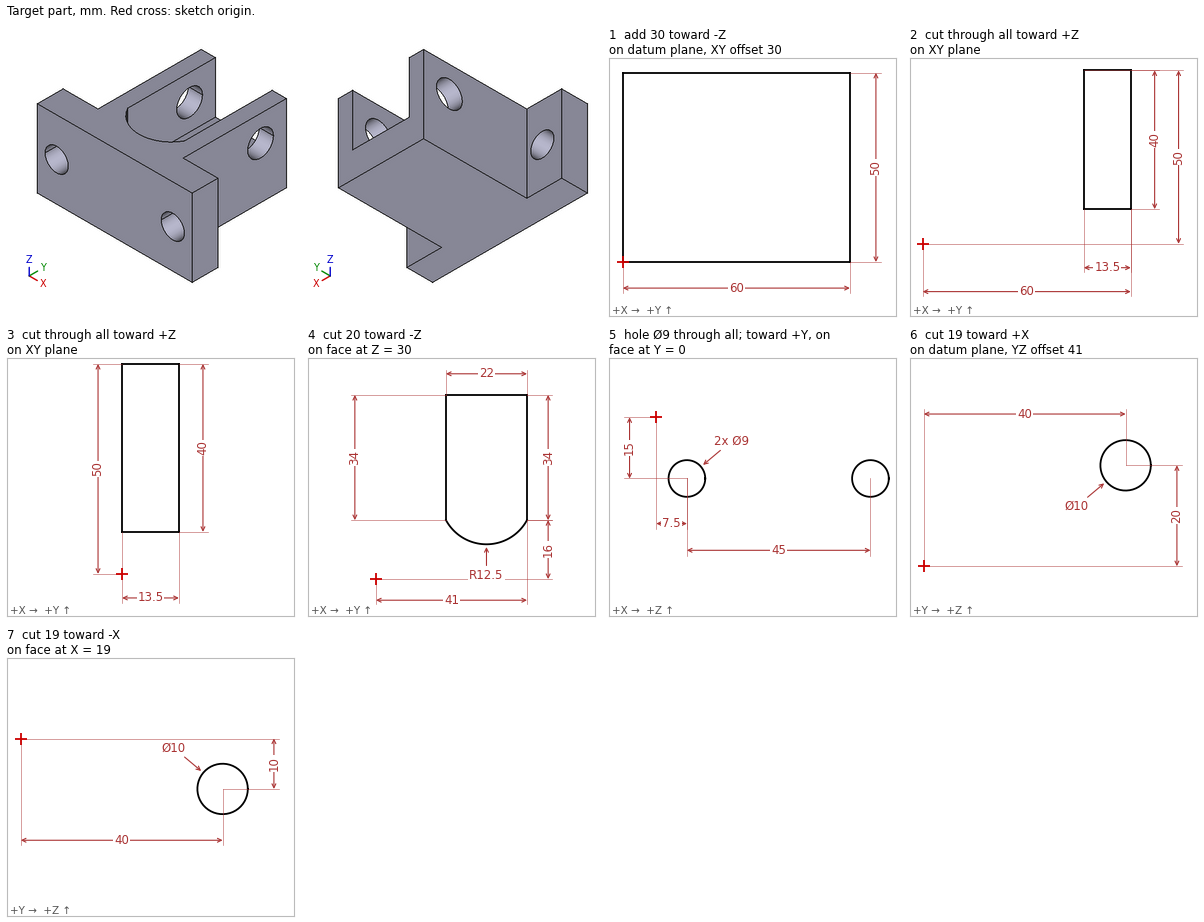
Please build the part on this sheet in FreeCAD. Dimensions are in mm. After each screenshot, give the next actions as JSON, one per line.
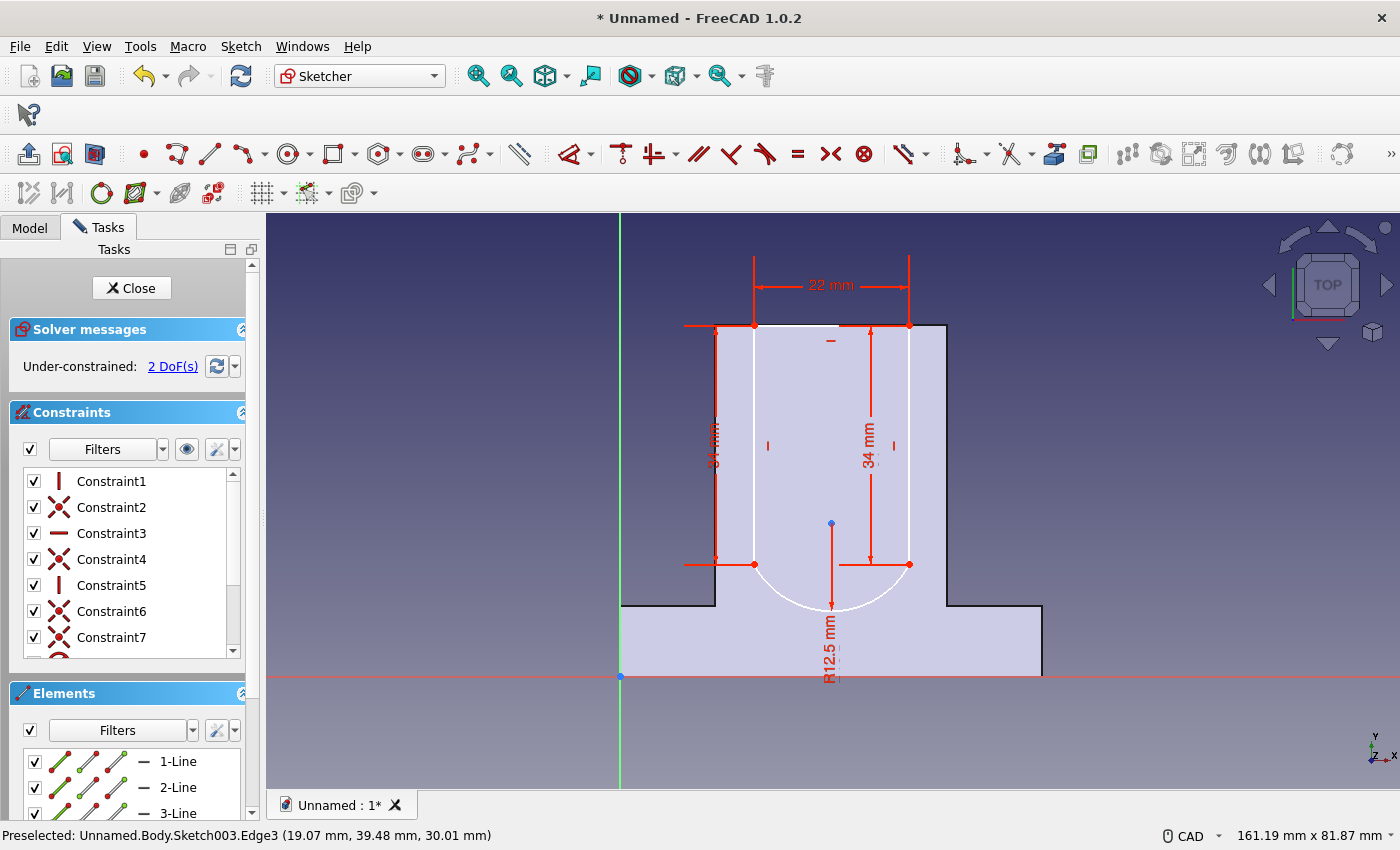
{"action": "left_click", "coordinate": [909, 565]}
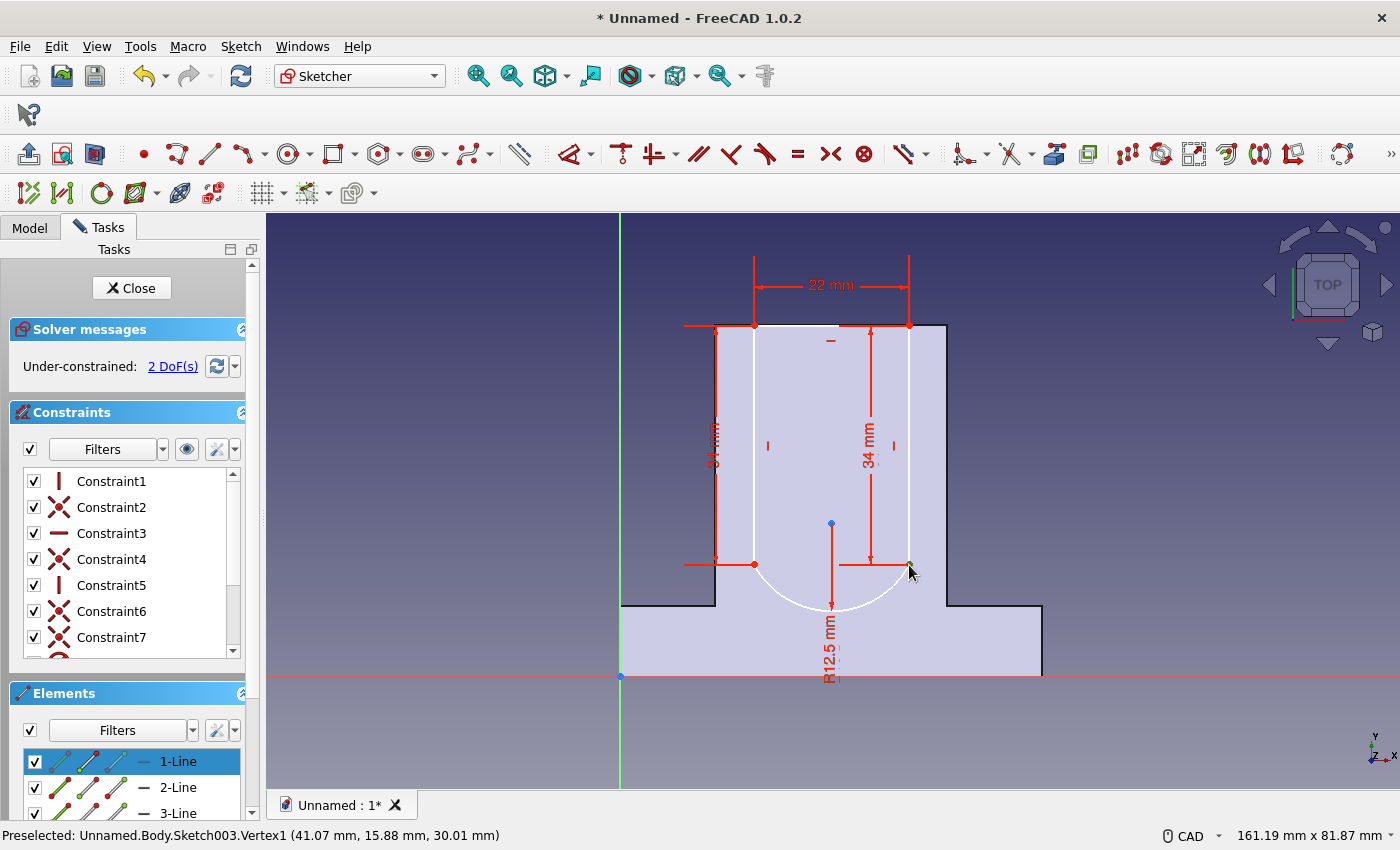
{"action": "key", "text": "l"}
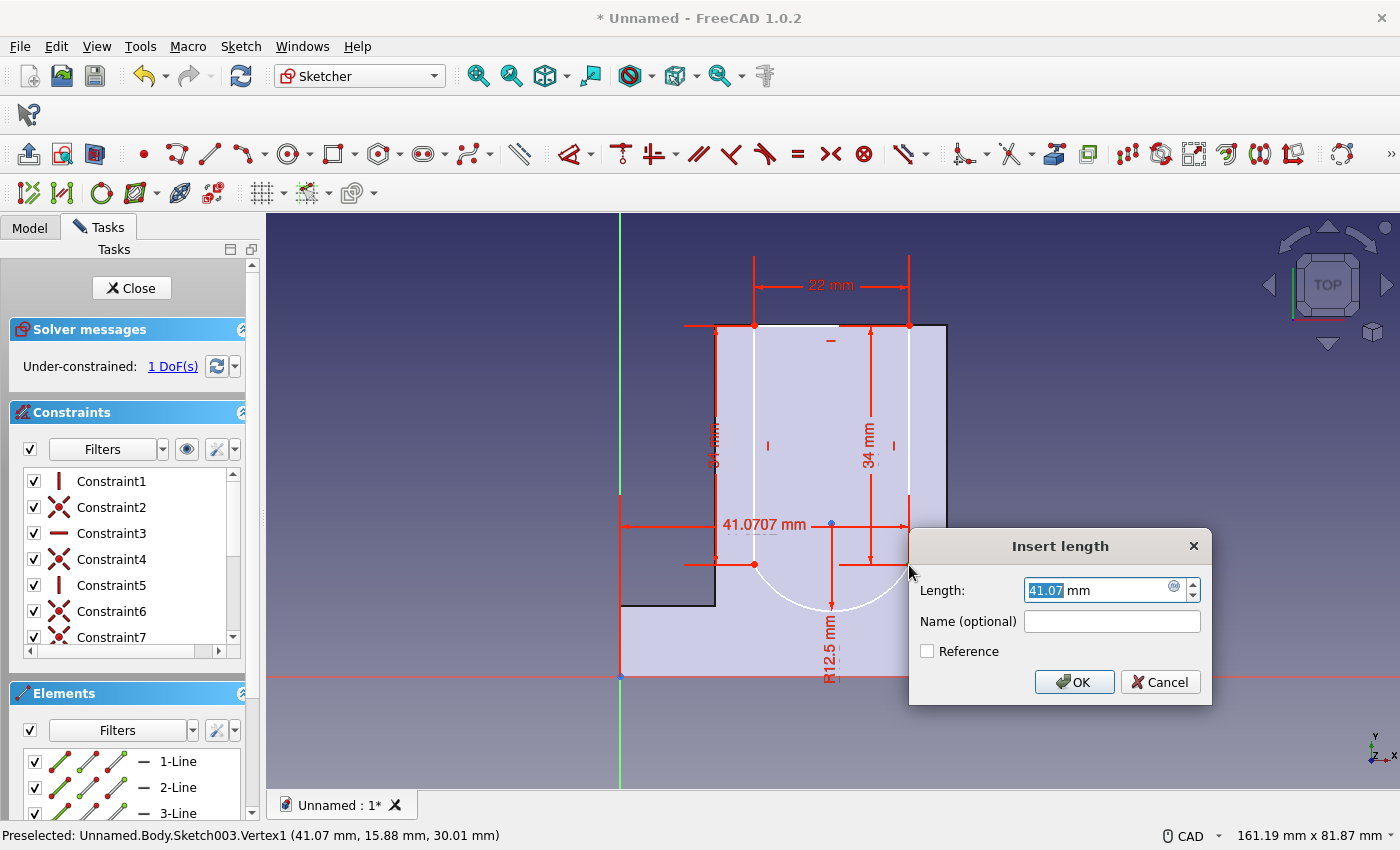
{"action": "type", "text": "41"}
{"action": "key", "text": "Return"}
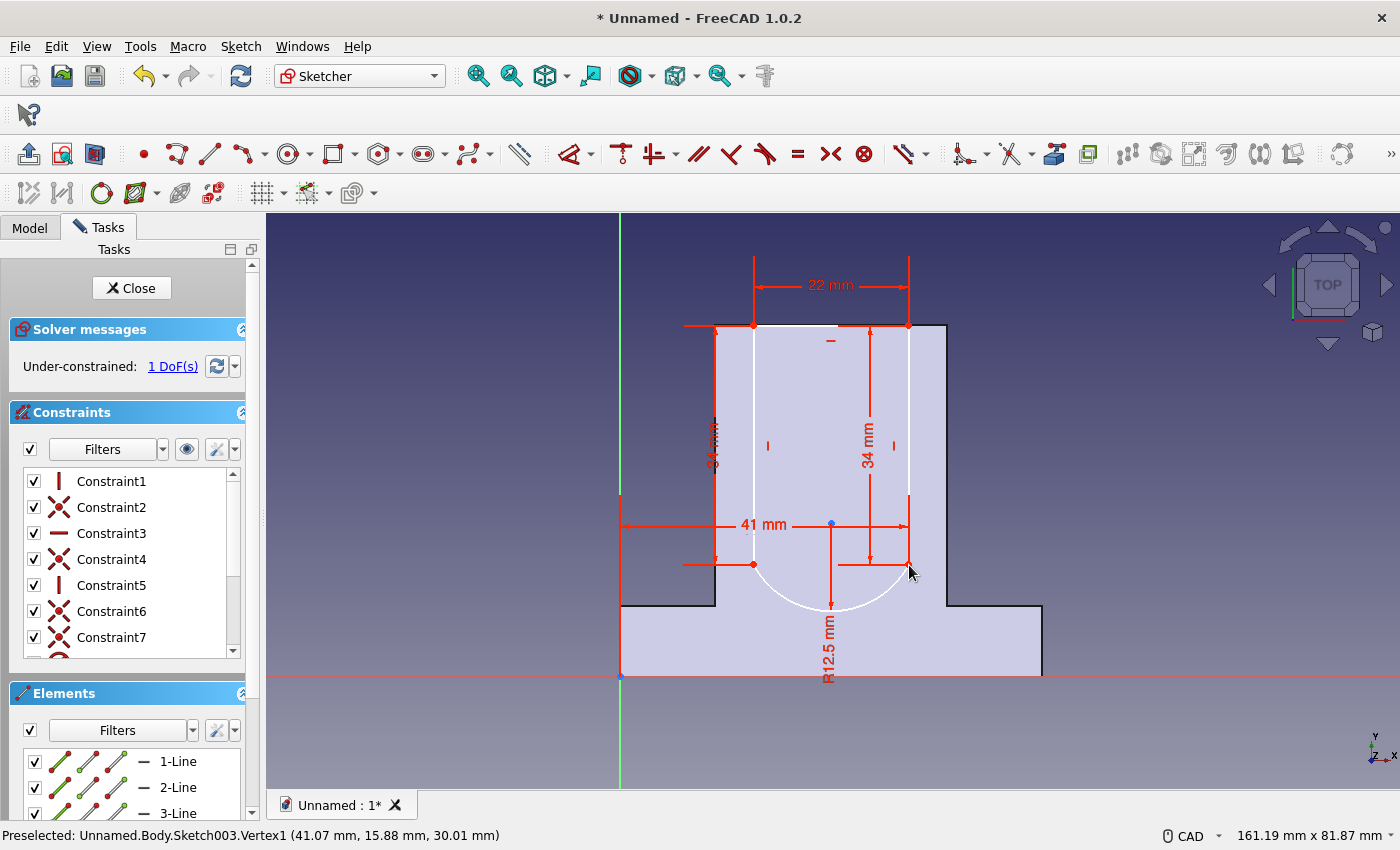
{"action": "left_click", "coordinate": [909, 565]}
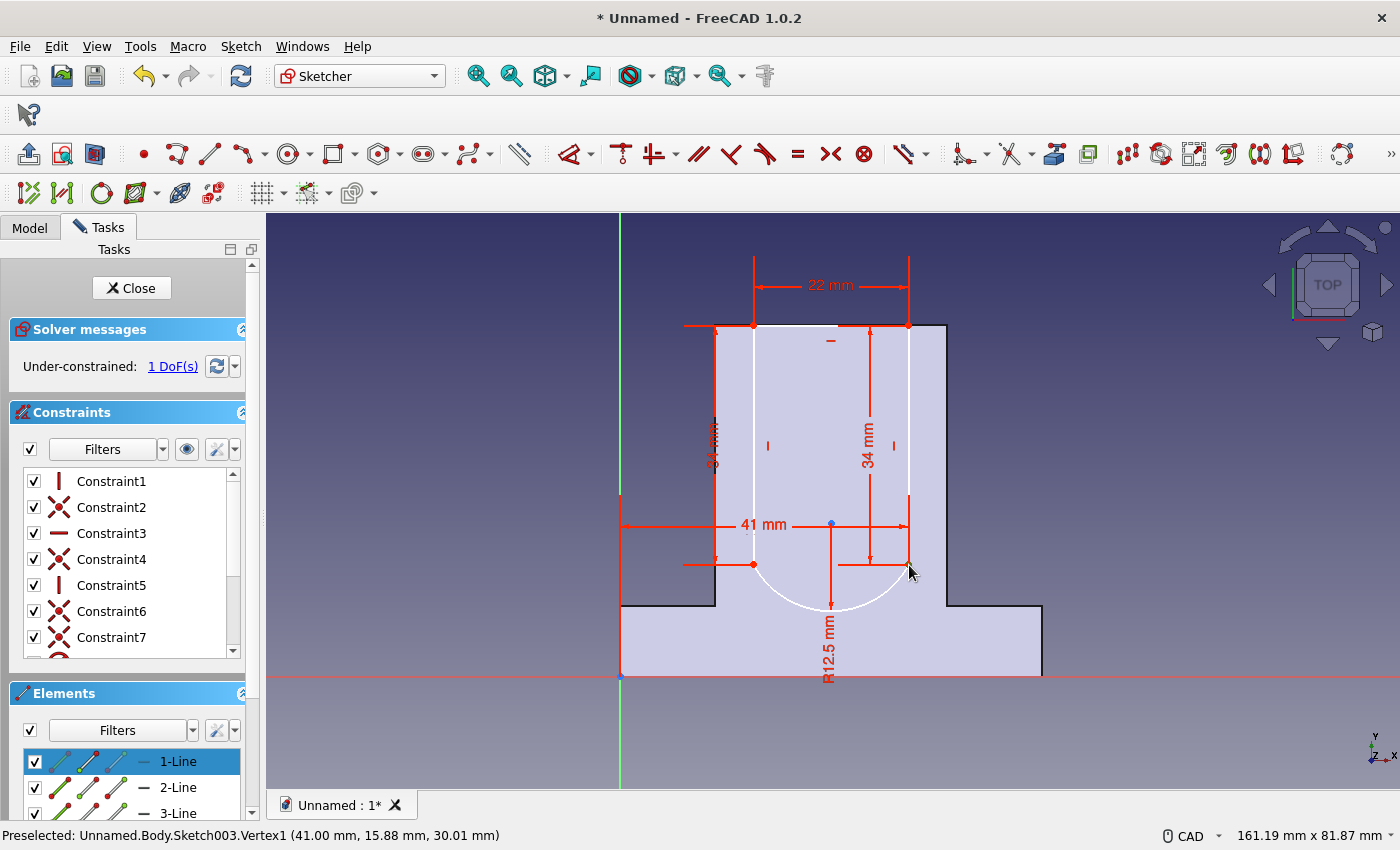
{"action": "key", "text": "i"}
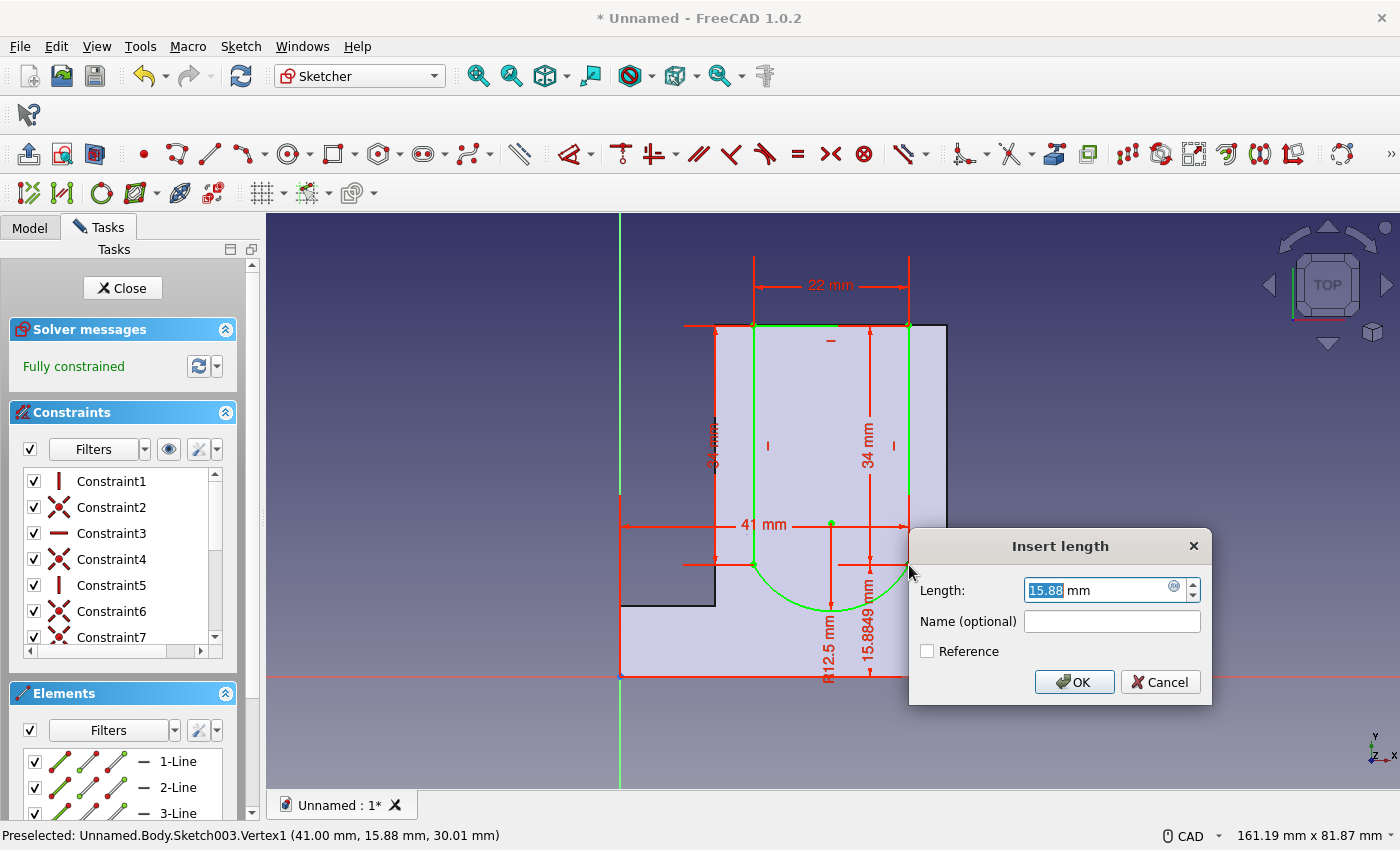
{"action": "type", "text": "16"}
{"action": "key", "text": "Return"}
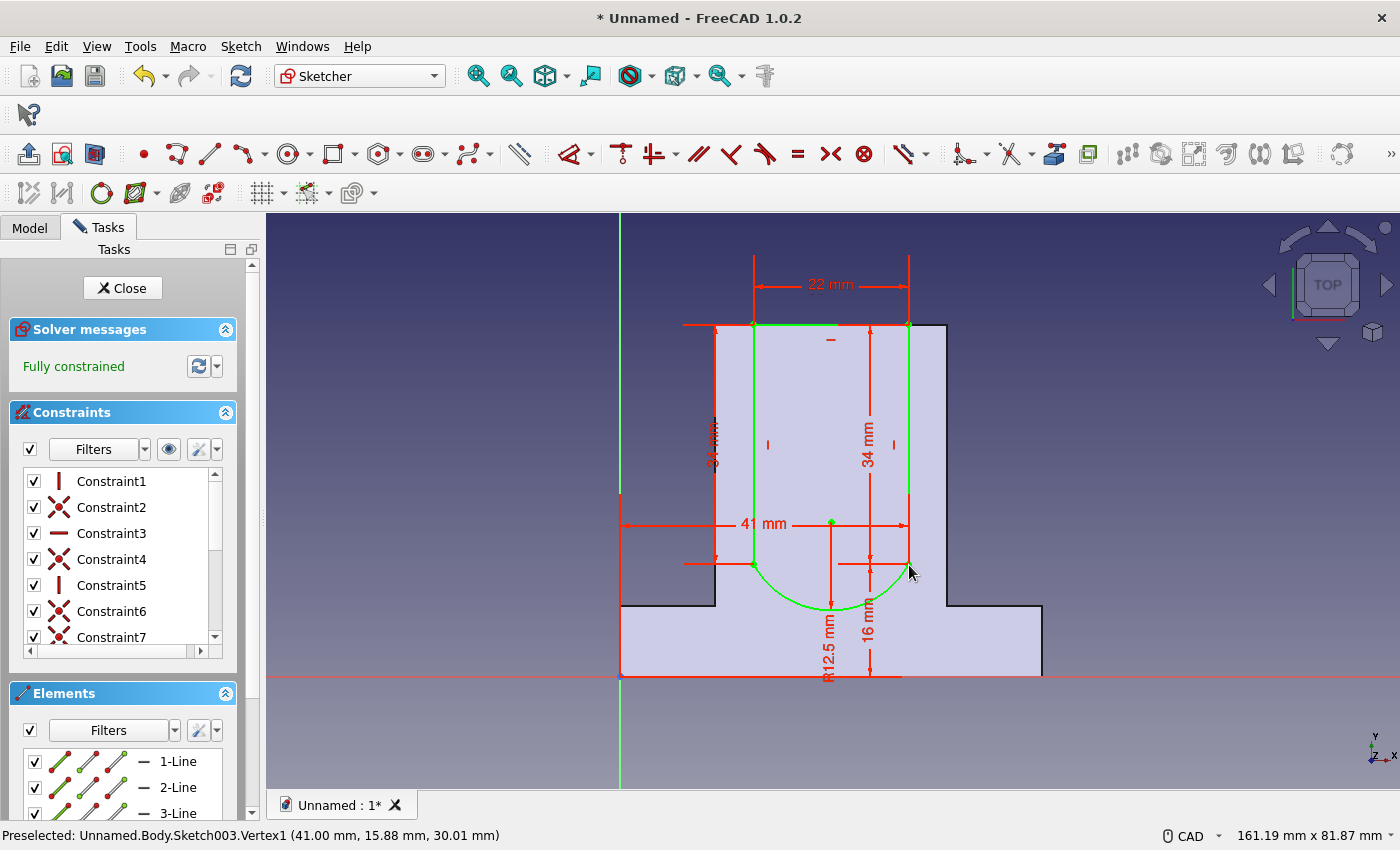
{"action": "left_click", "coordinate": [123, 288]}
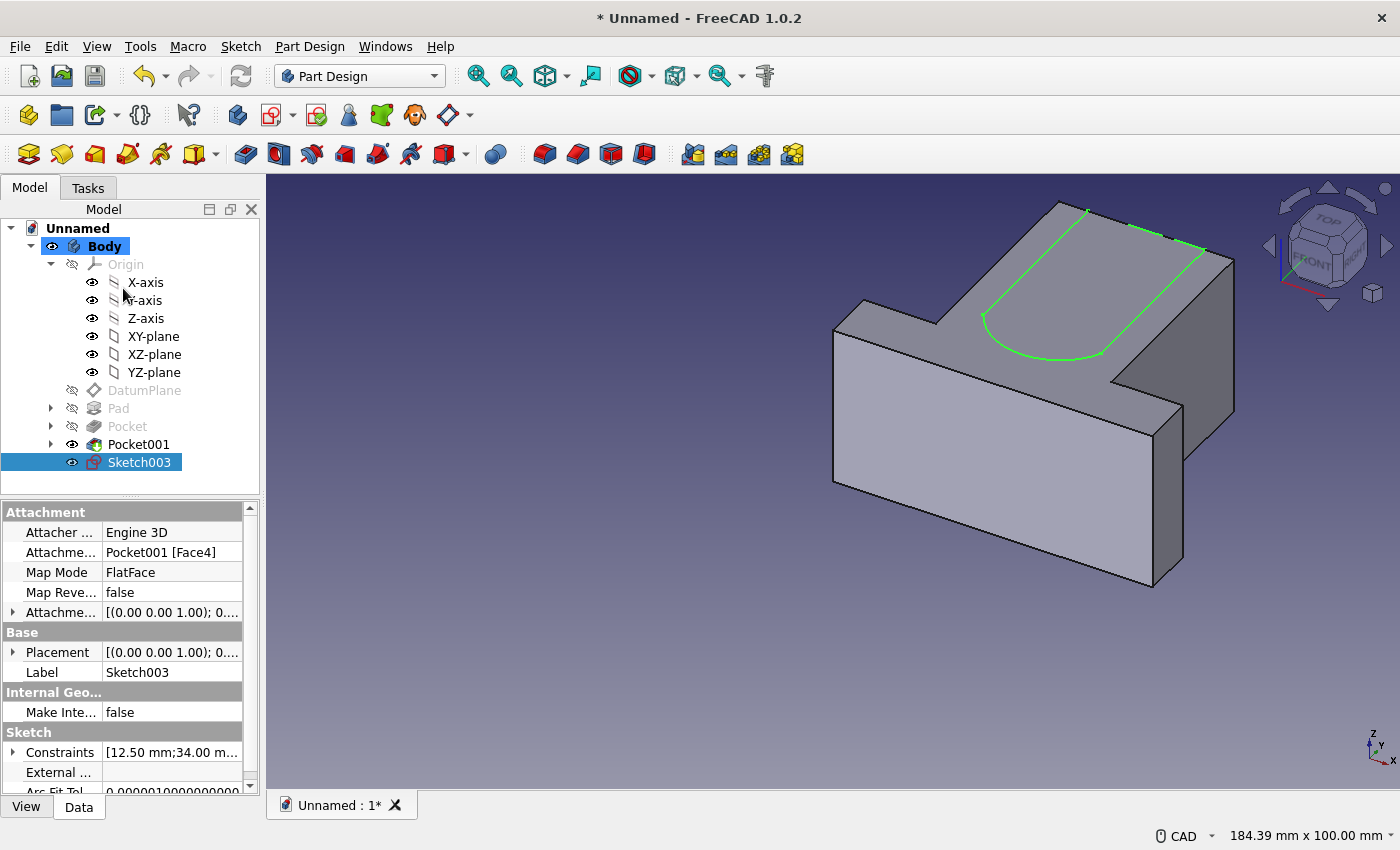
{"action": "left_click", "coordinate": [246, 154]}